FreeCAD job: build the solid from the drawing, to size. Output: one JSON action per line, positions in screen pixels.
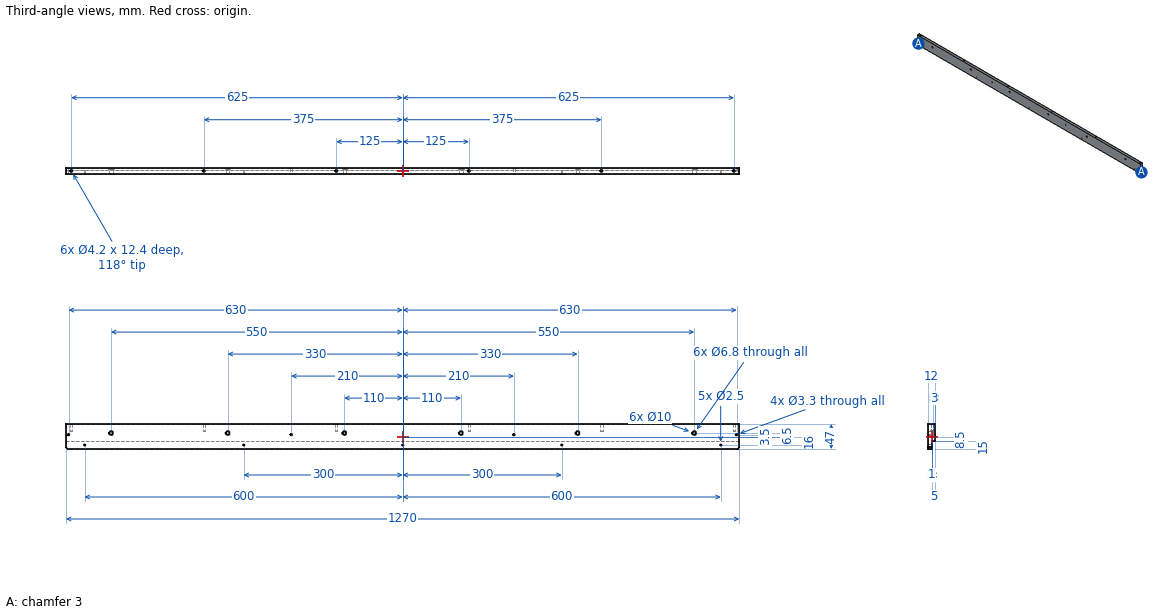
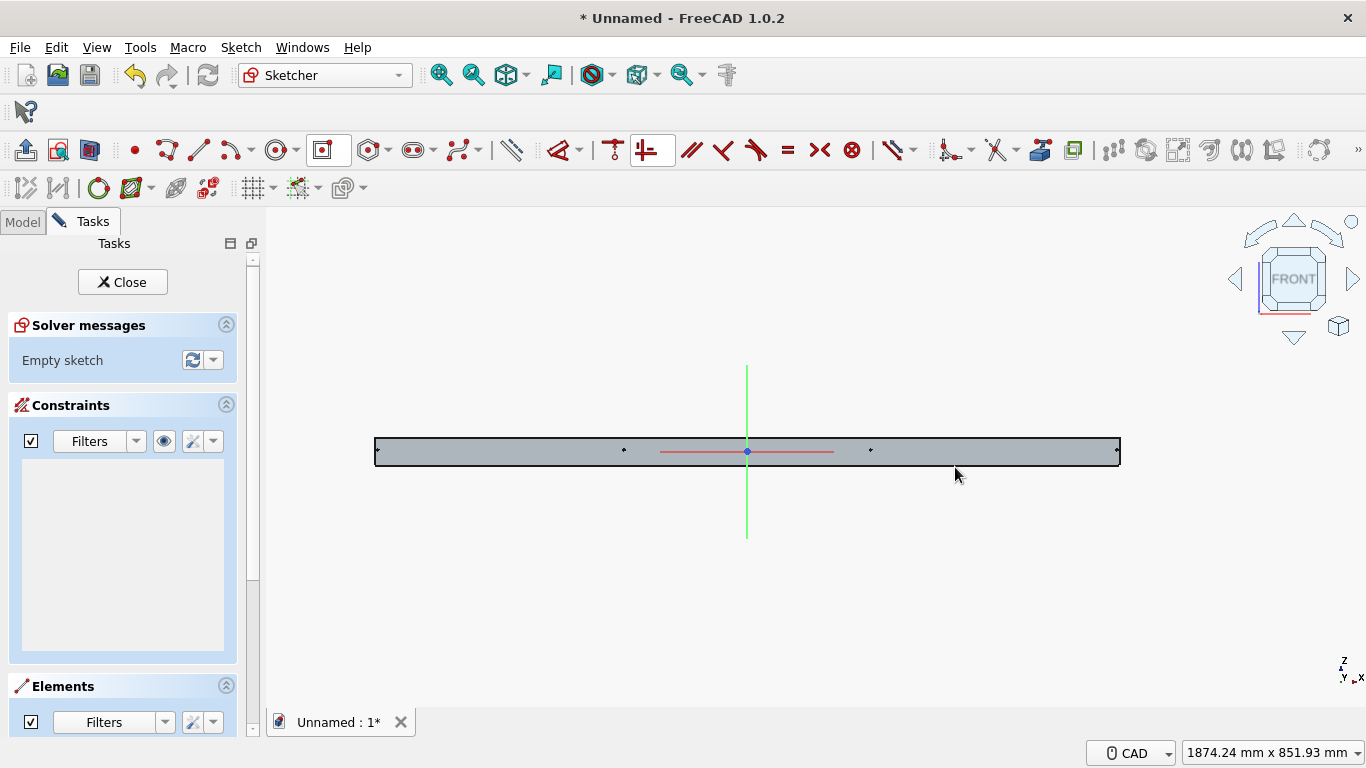
{"action": "left_click", "coordinate": [276, 150]}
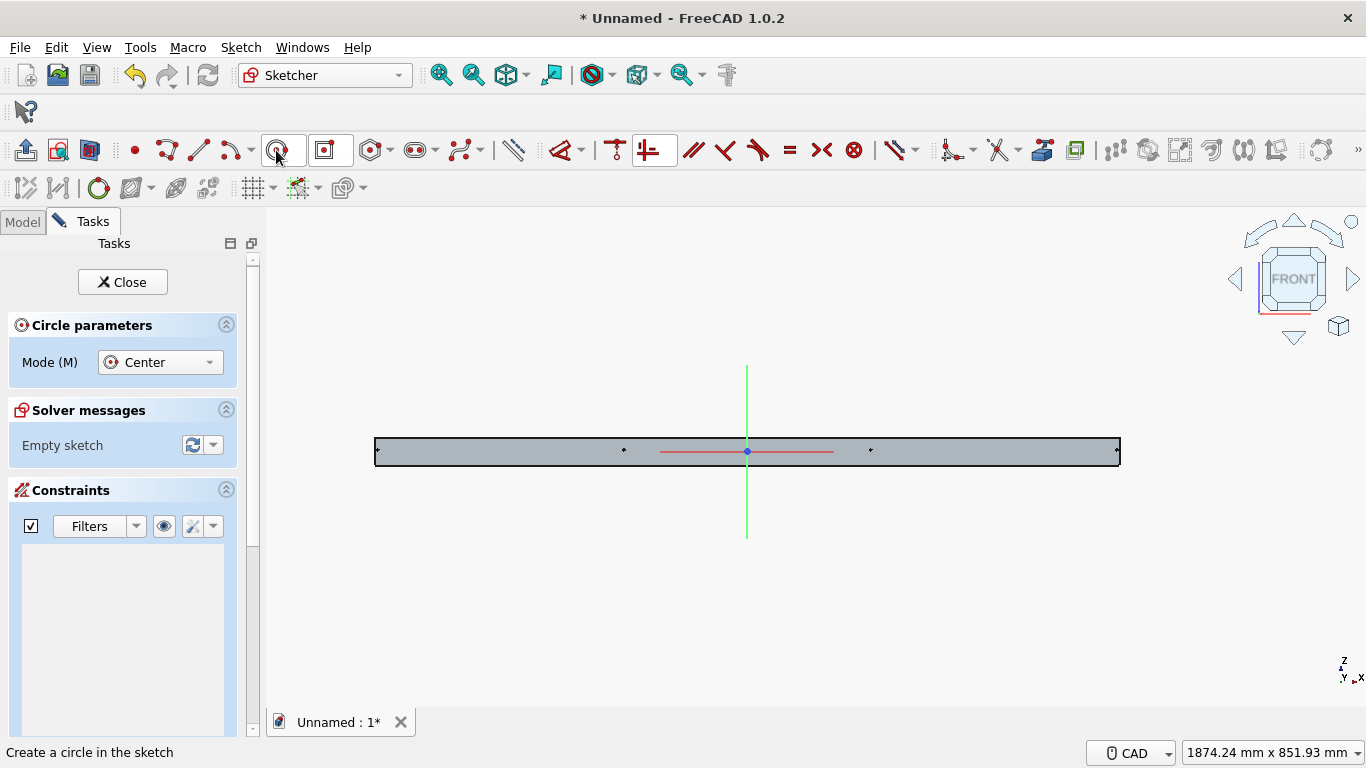
{"action": "scroll", "coordinate": [1099, 461], "scroll_direction": "up", "scroll_amount": 18}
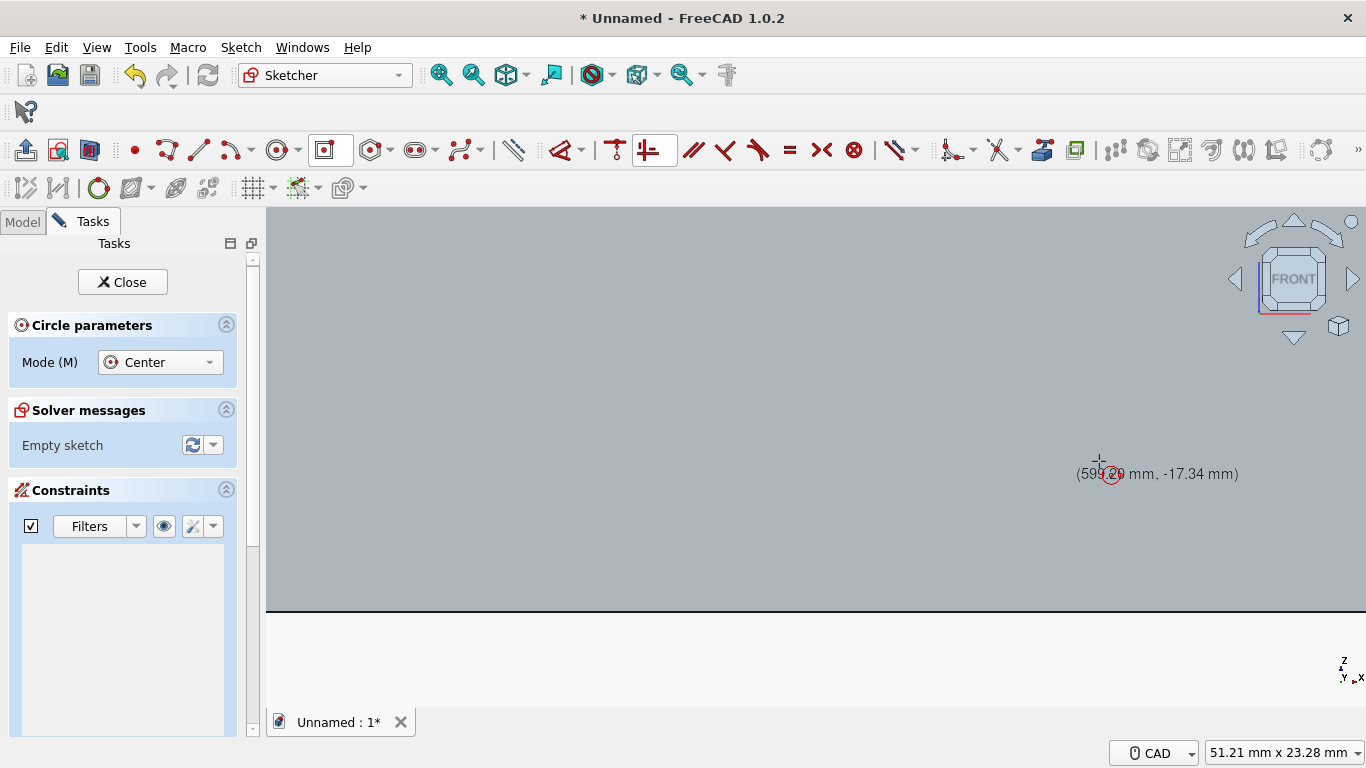
{"action": "scroll", "coordinate": [1100, 462], "scroll_direction": "down", "scroll_amount": 18}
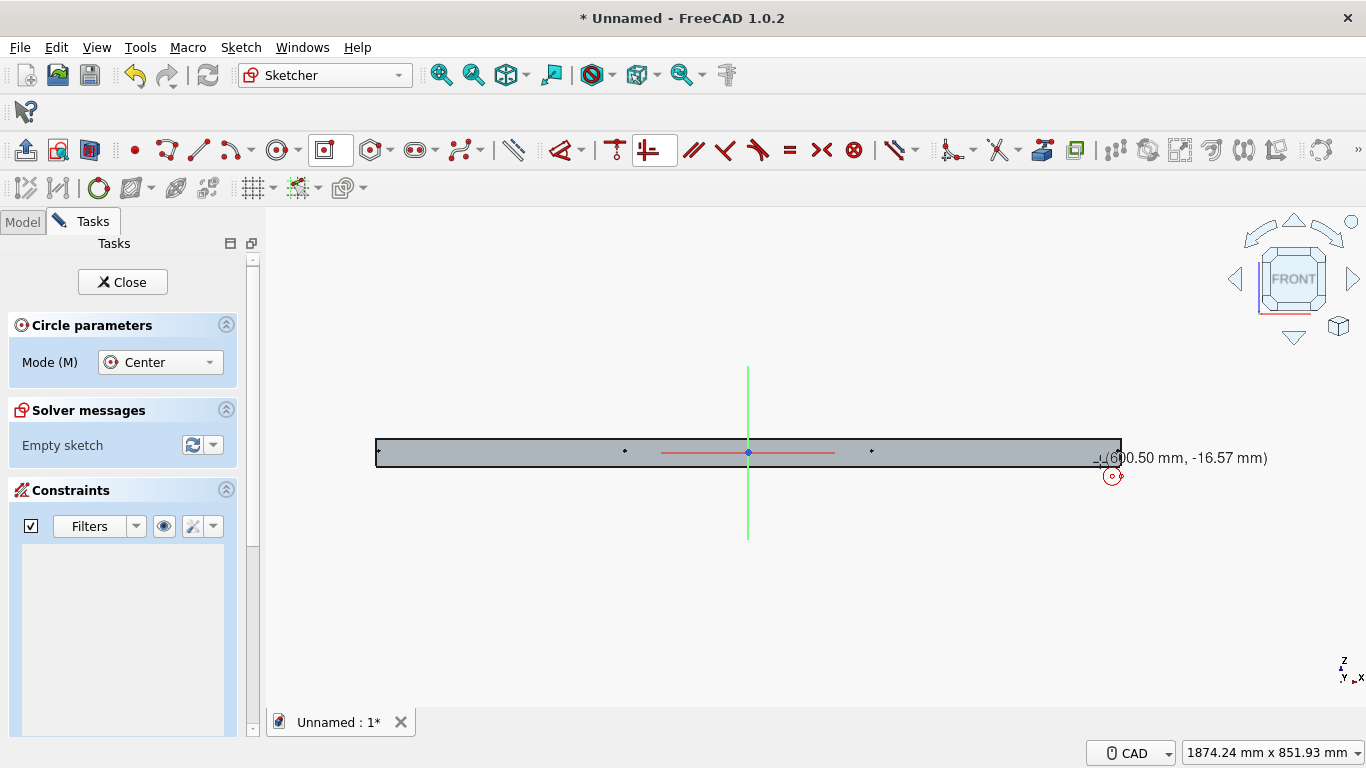
{"action": "scroll", "coordinate": [1100, 462], "scroll_direction": "up", "scroll_amount": 3}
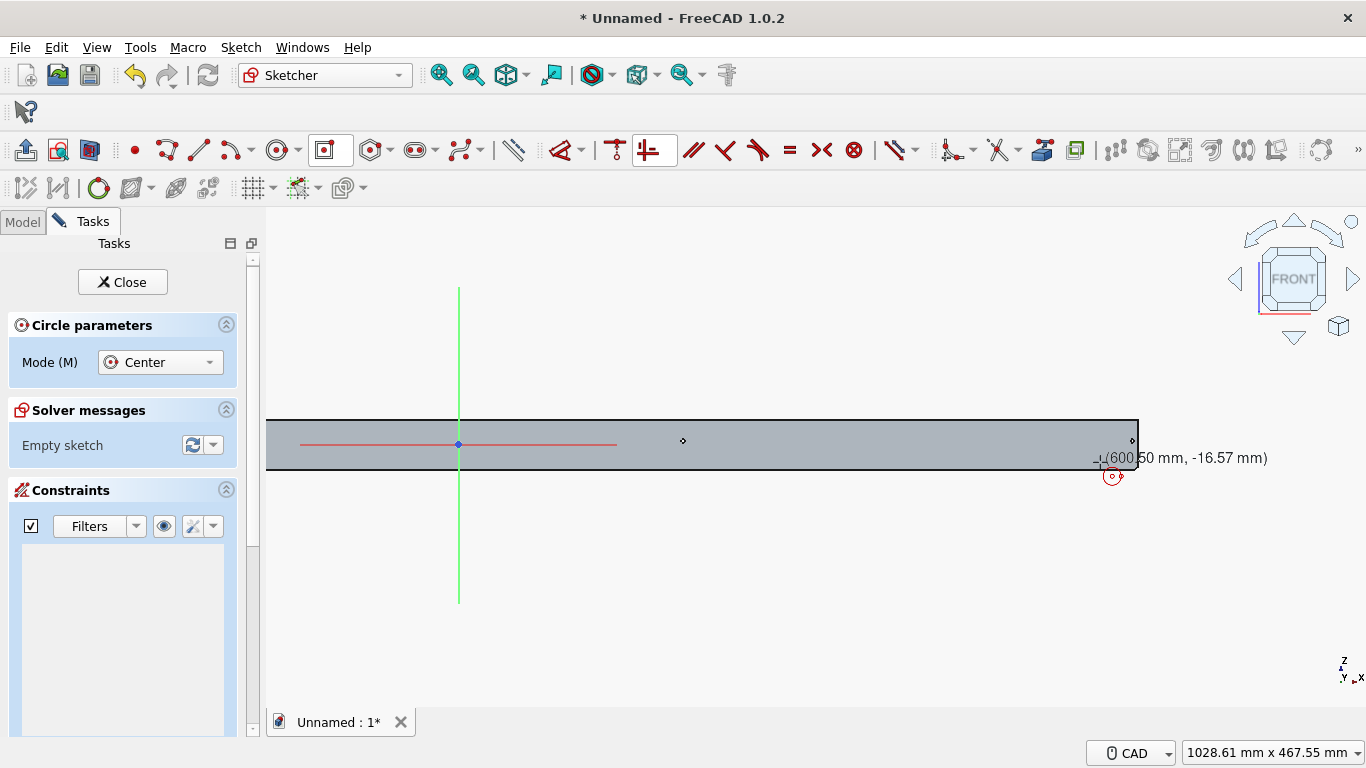
{"action": "left_click", "coordinate": [1100, 462]}
{"action": "mouse_move", "coordinate": [1101, 461]}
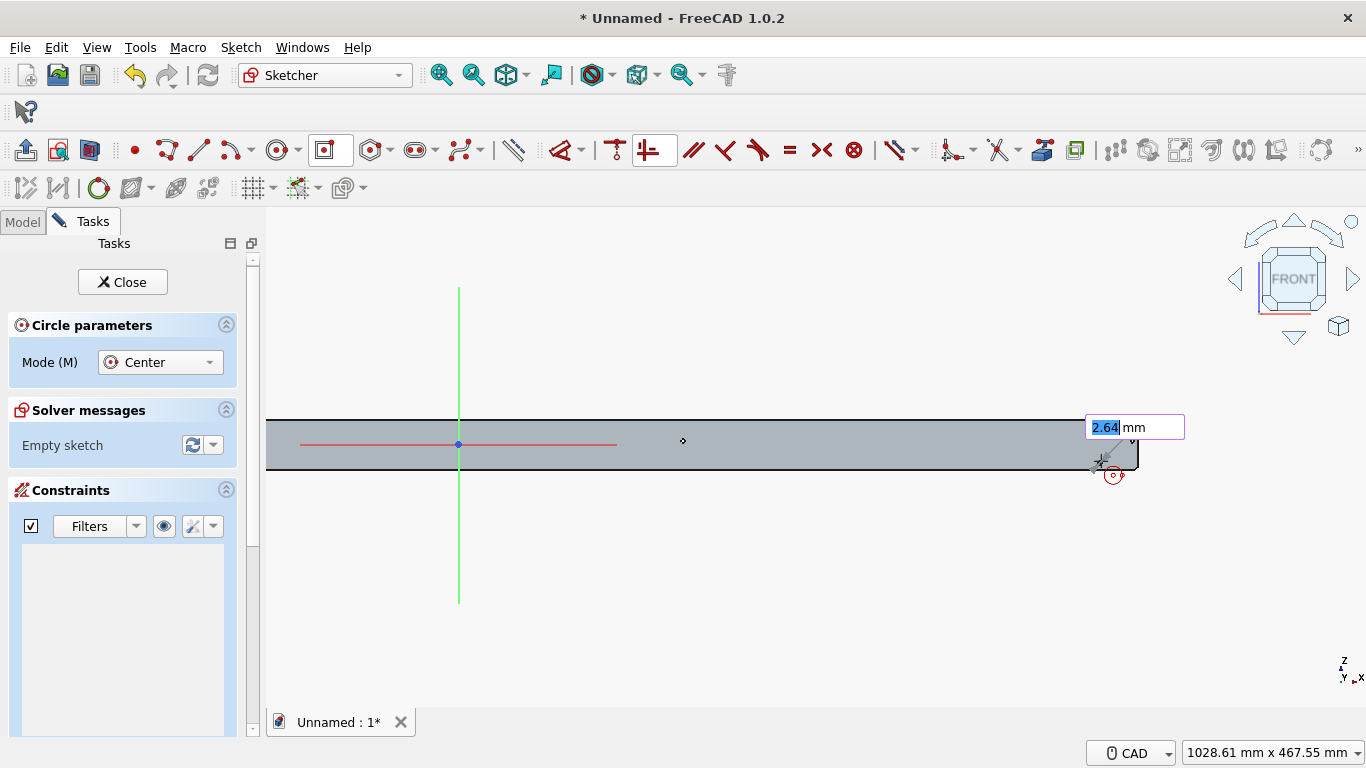
{"action": "type", "text": "2.5"}
{"action": "key", "text": "Return"}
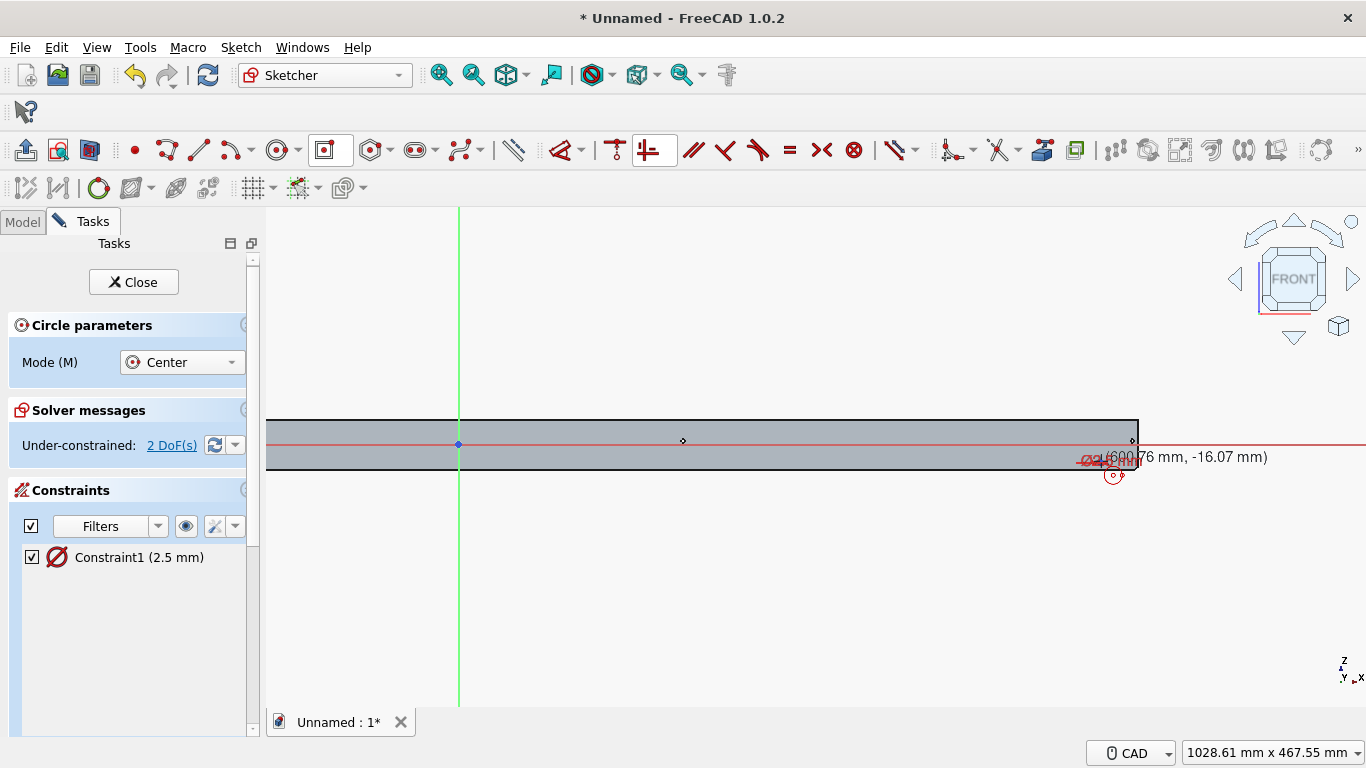
{"action": "scroll", "coordinate": [779, 462], "scroll_direction": "up", "scroll_amount": 15}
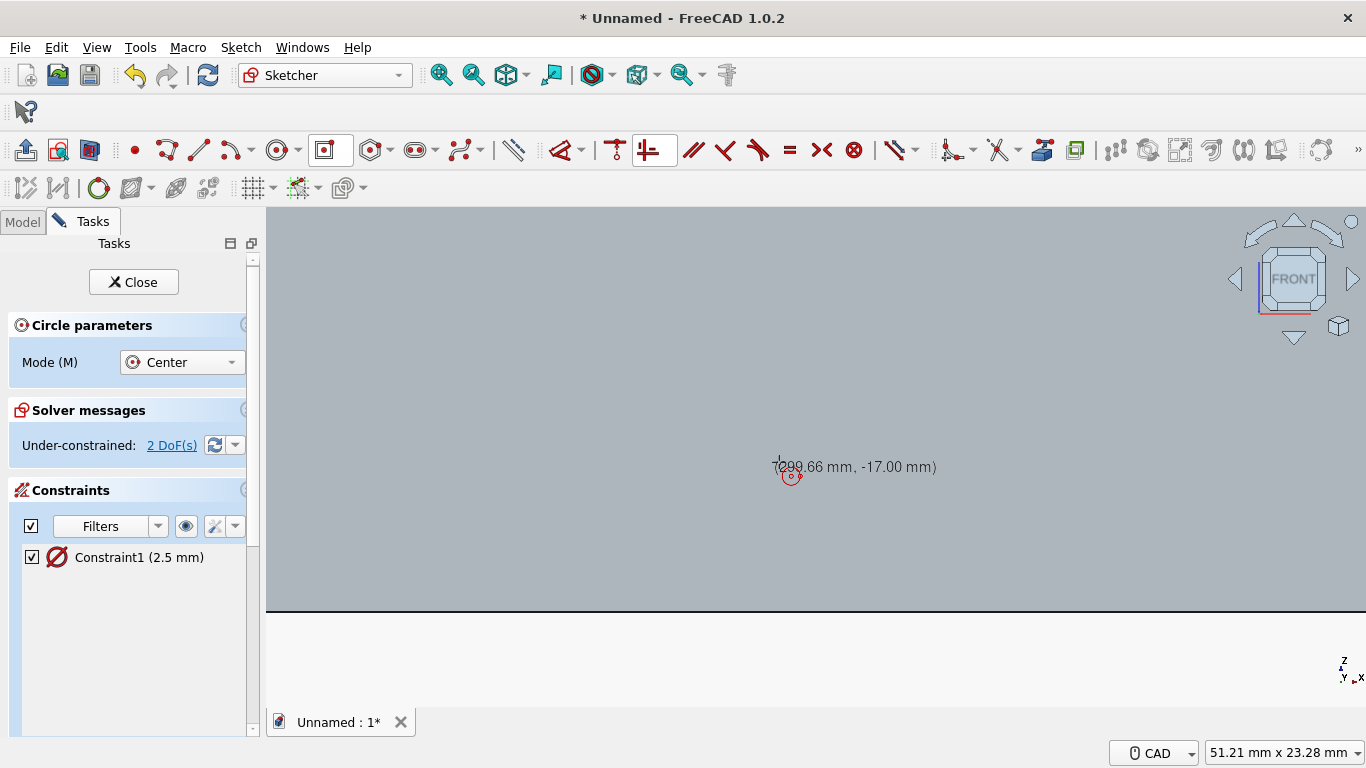
{"action": "scroll", "coordinate": [928, 462], "scroll_direction": "down", "scroll_amount": 18}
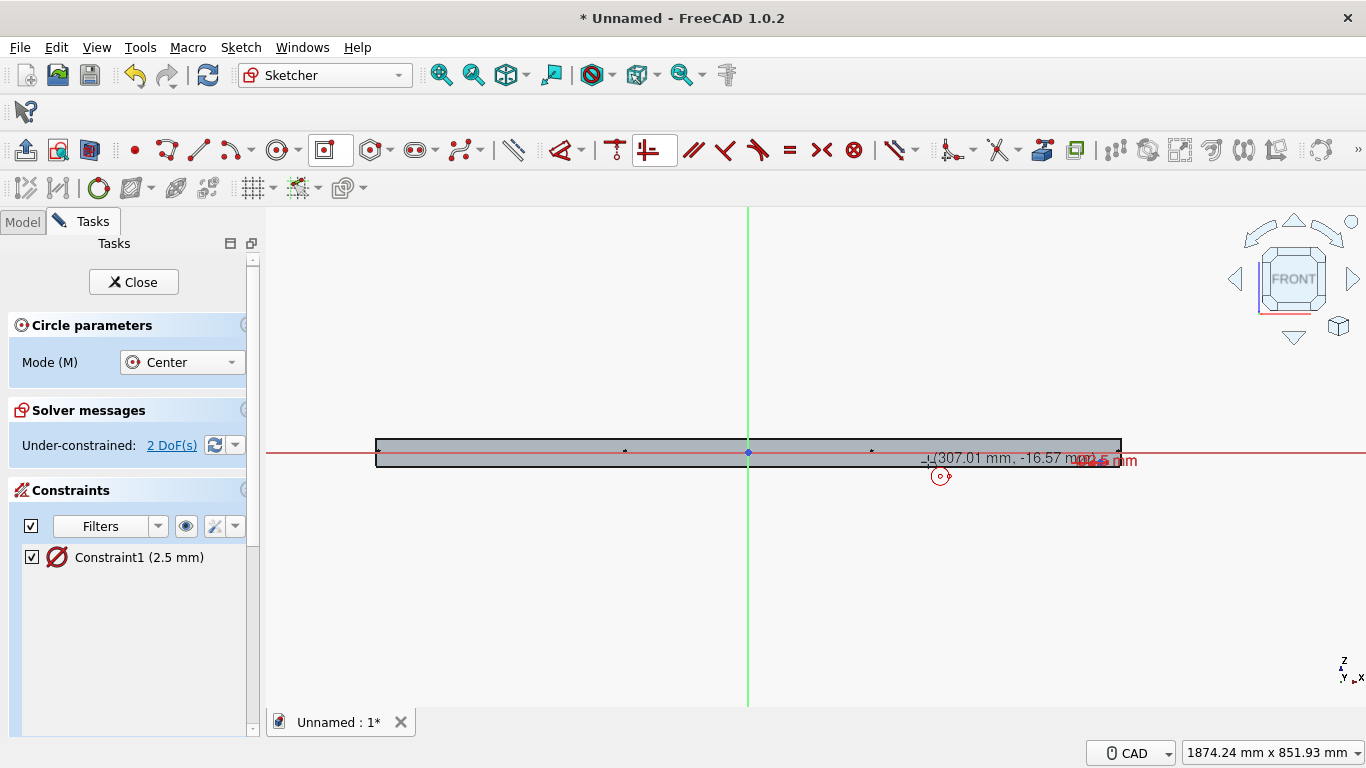
{"action": "scroll", "coordinate": [924, 462], "scroll_direction": "up", "scroll_amount": 3}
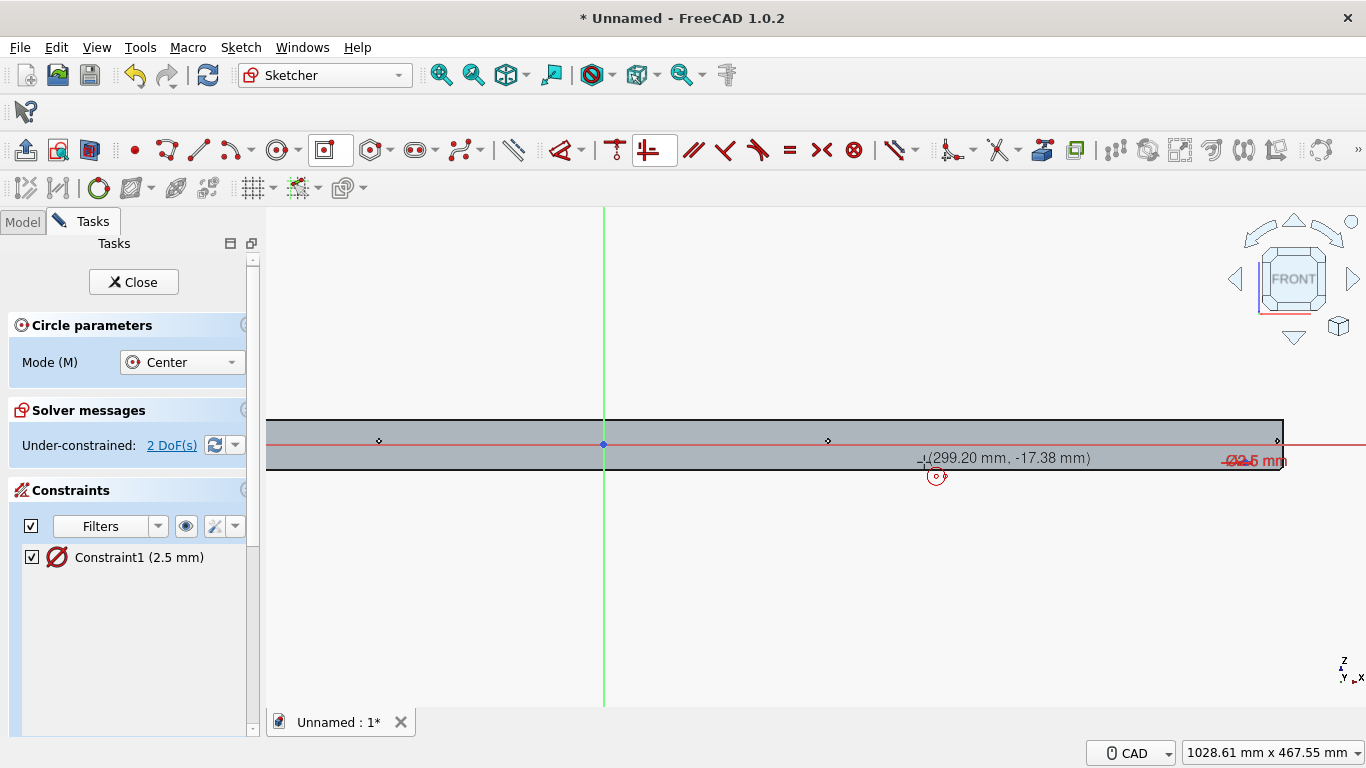
{"action": "left_click", "coordinate": [924, 462]}
{"action": "mouse_move", "coordinate": [925, 461]}